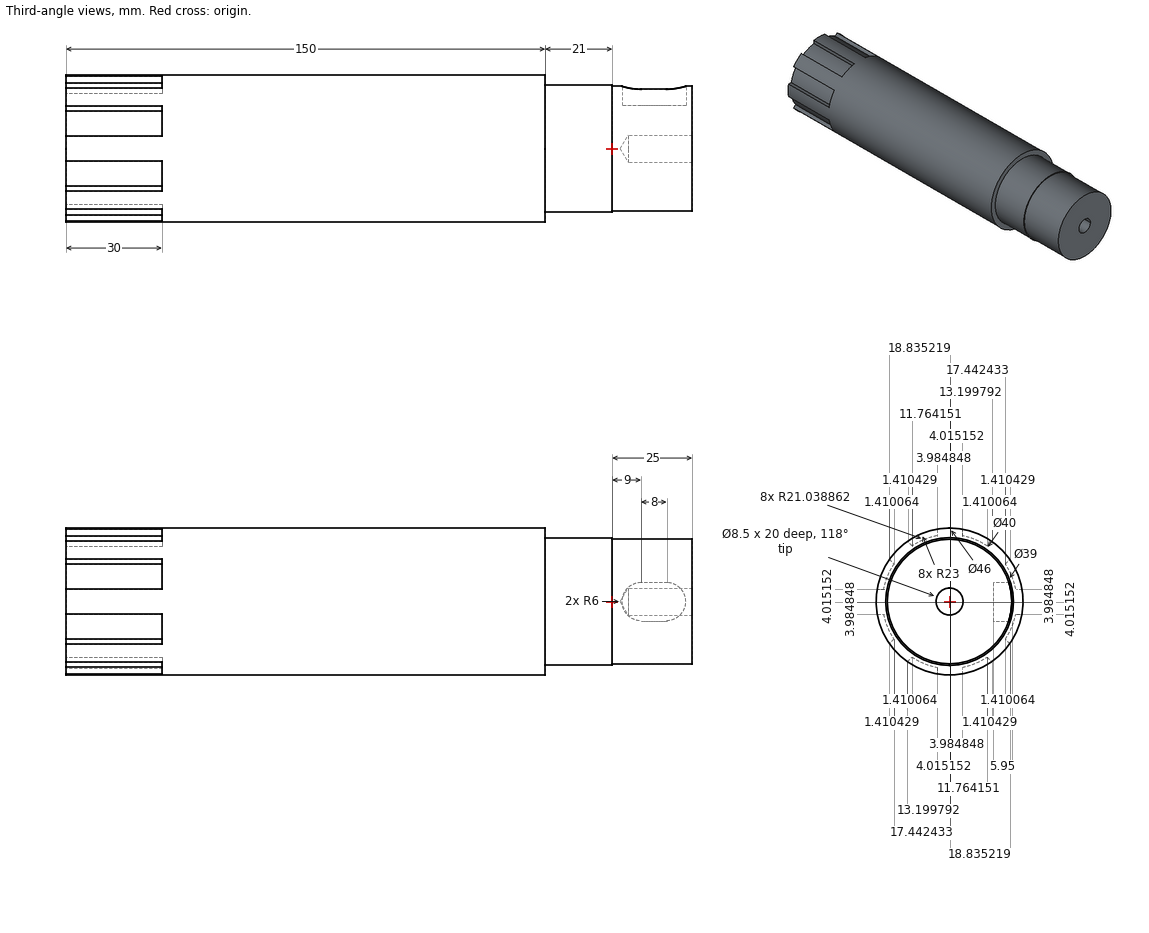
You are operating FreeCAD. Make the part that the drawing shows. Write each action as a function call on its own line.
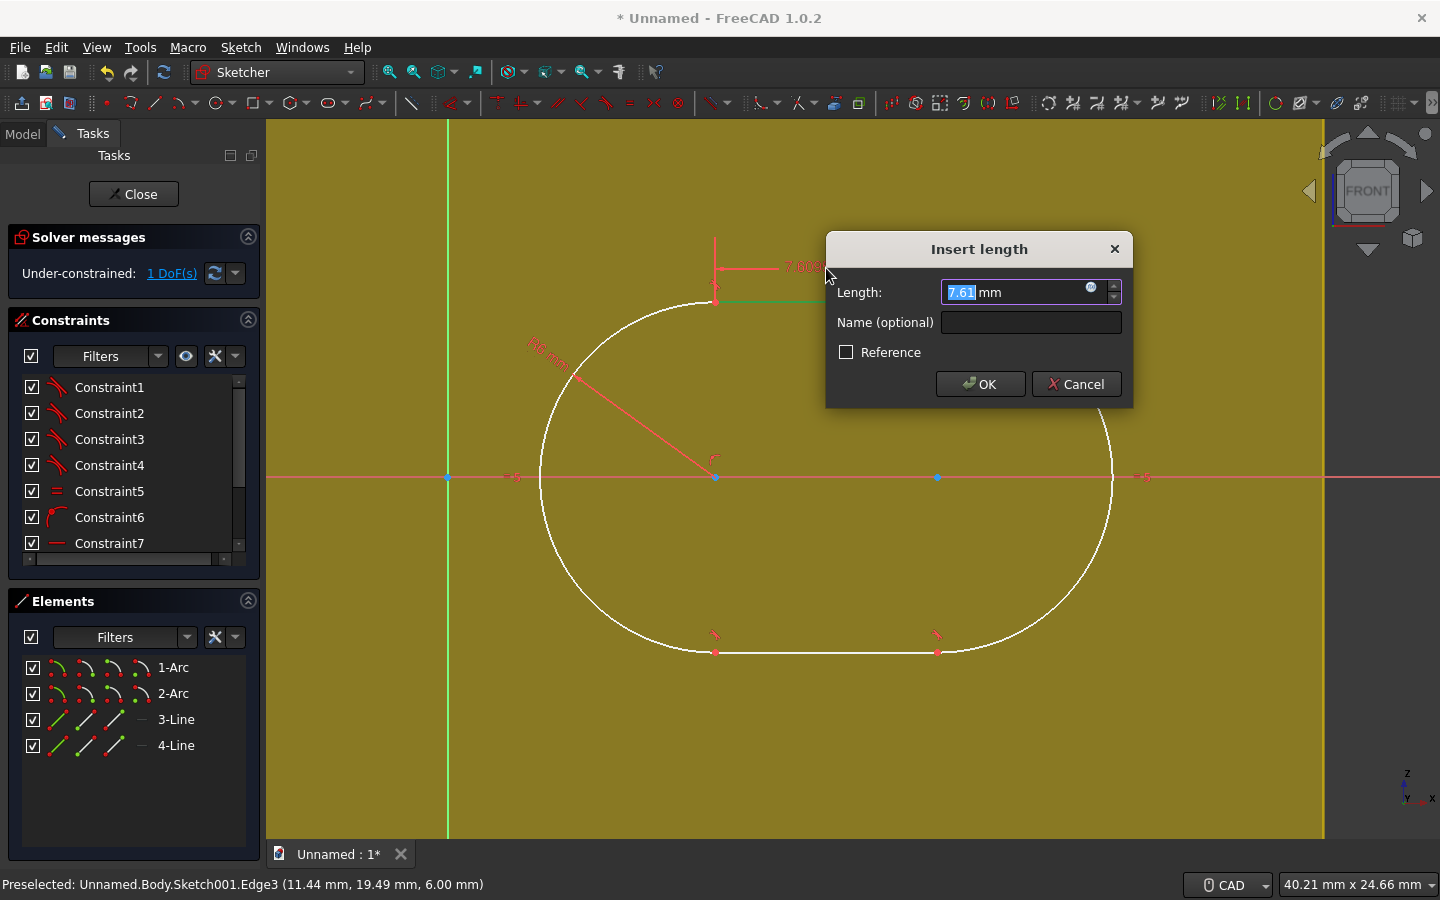
text(8)
key(Return)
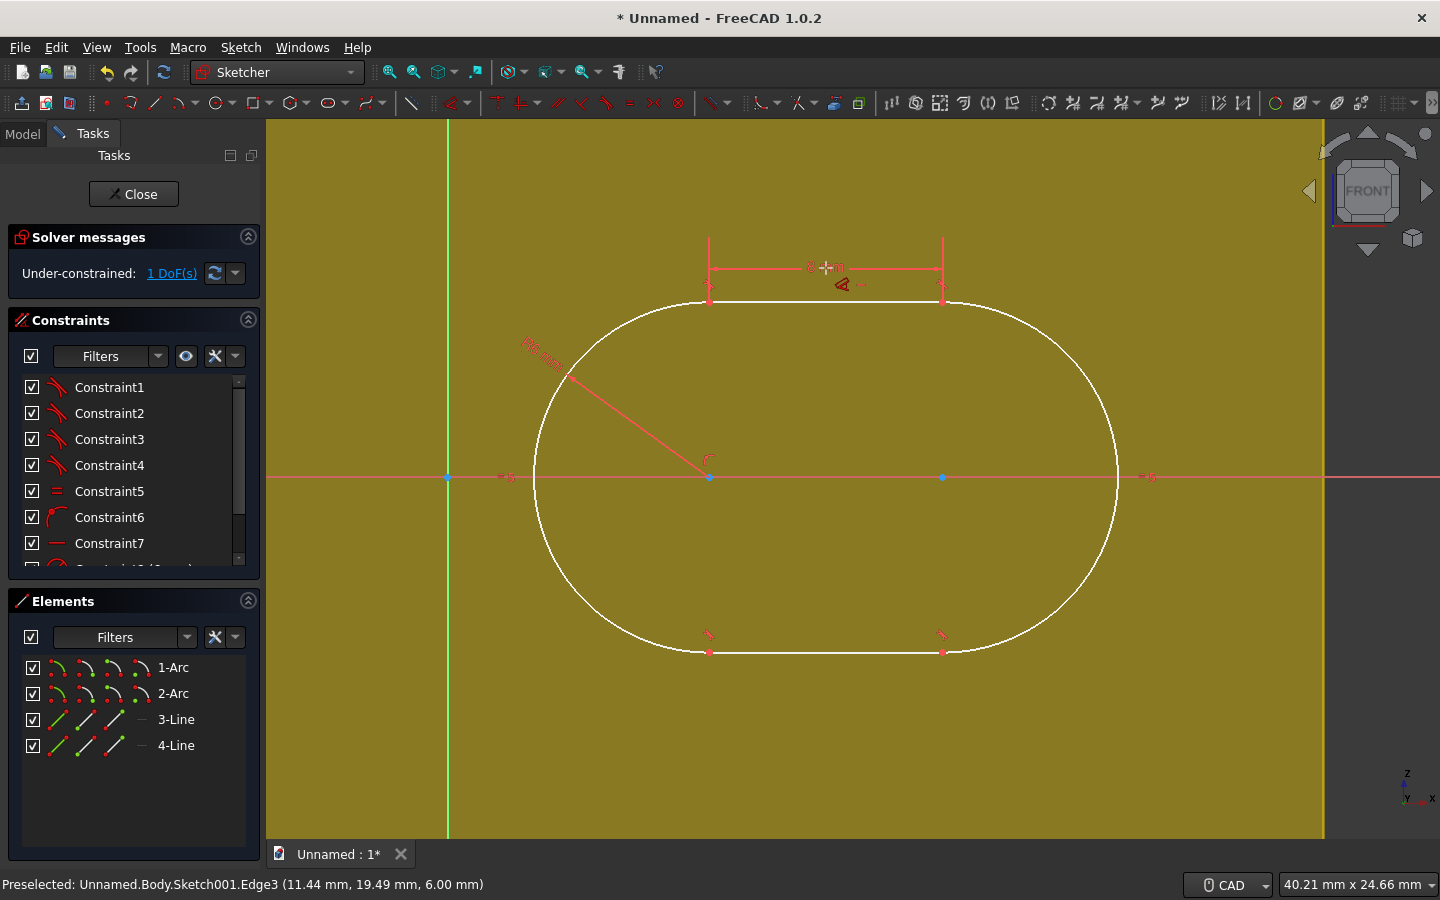
click(709, 302)
click(579, 268)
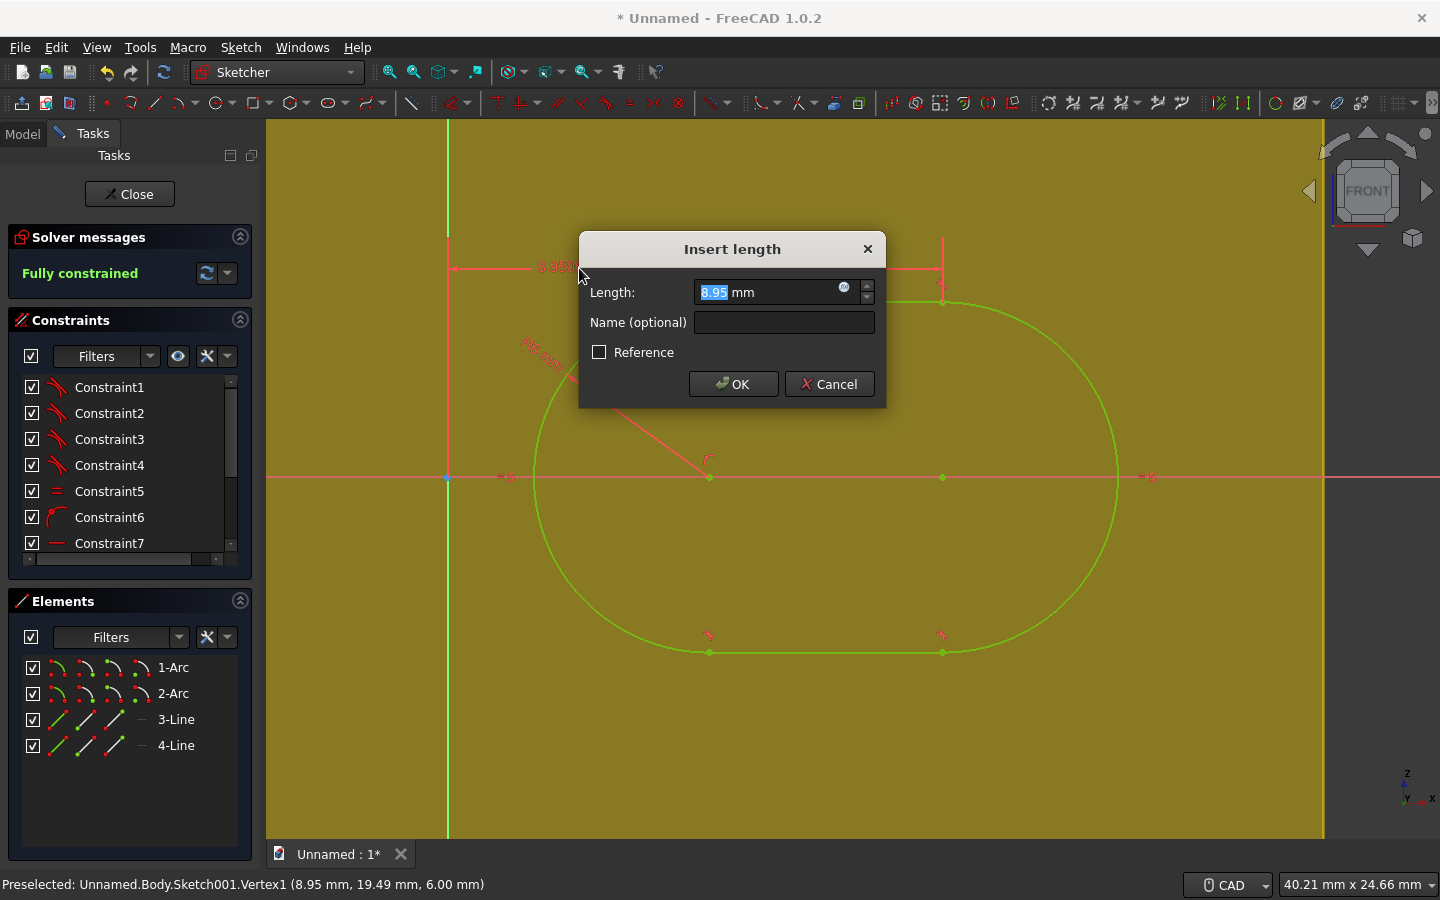
text(9)
key(Return)
key(Escape)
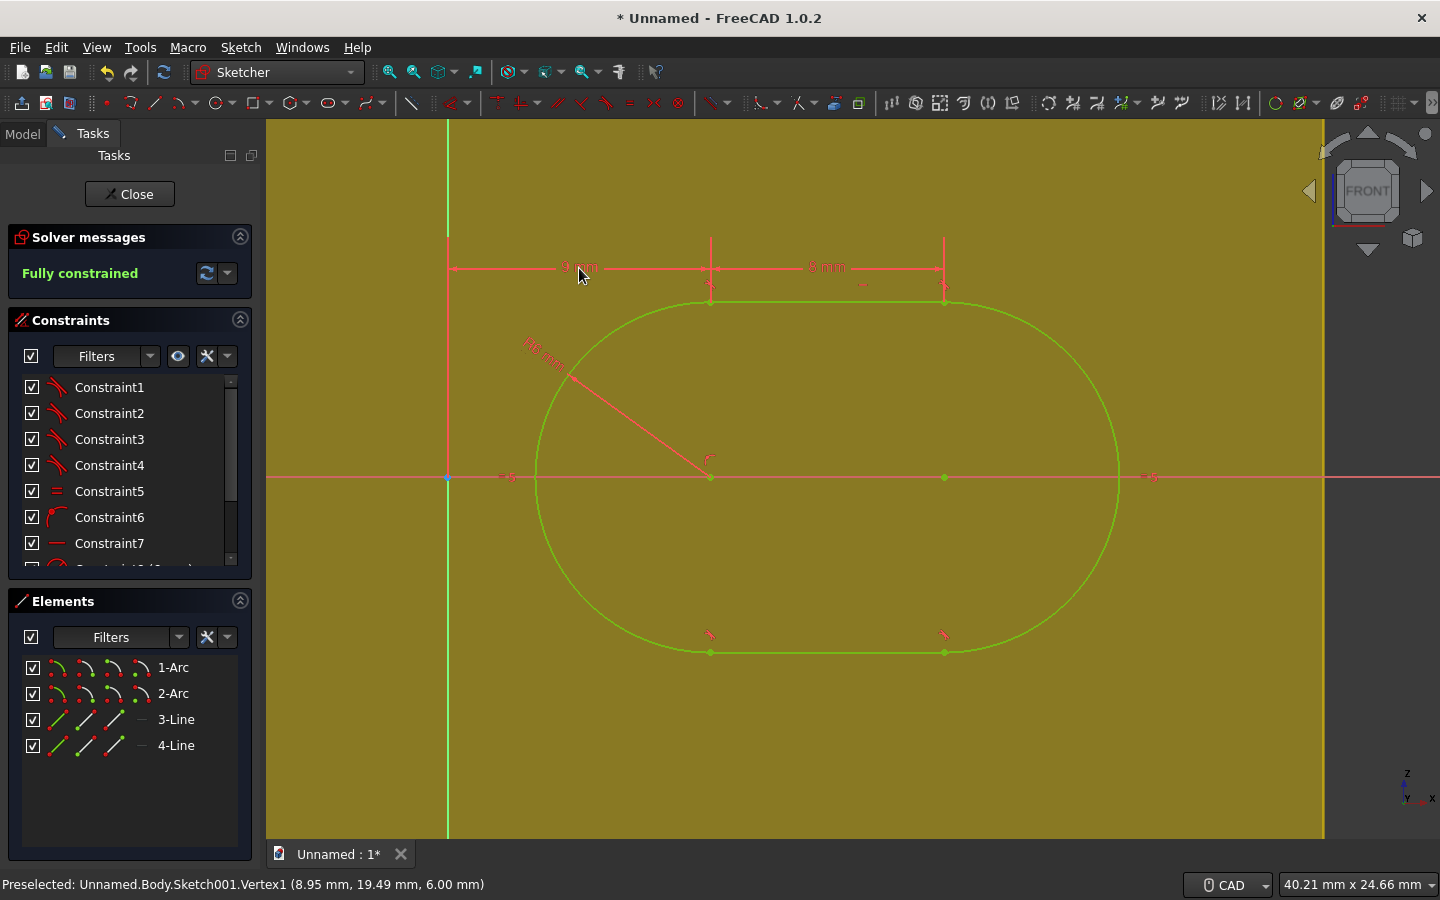
click(130, 194)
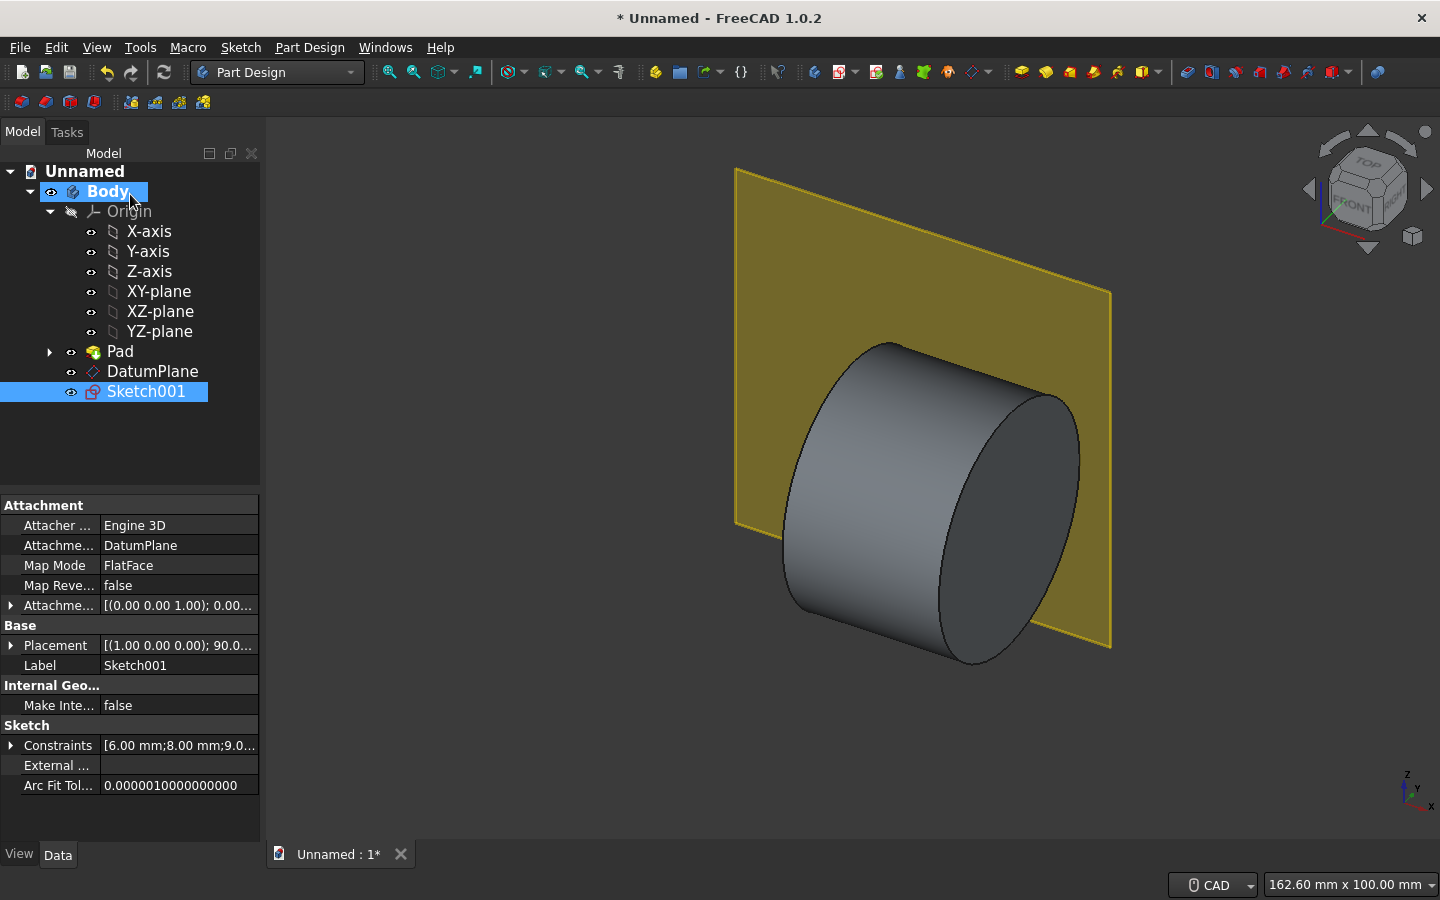
click(1188, 72)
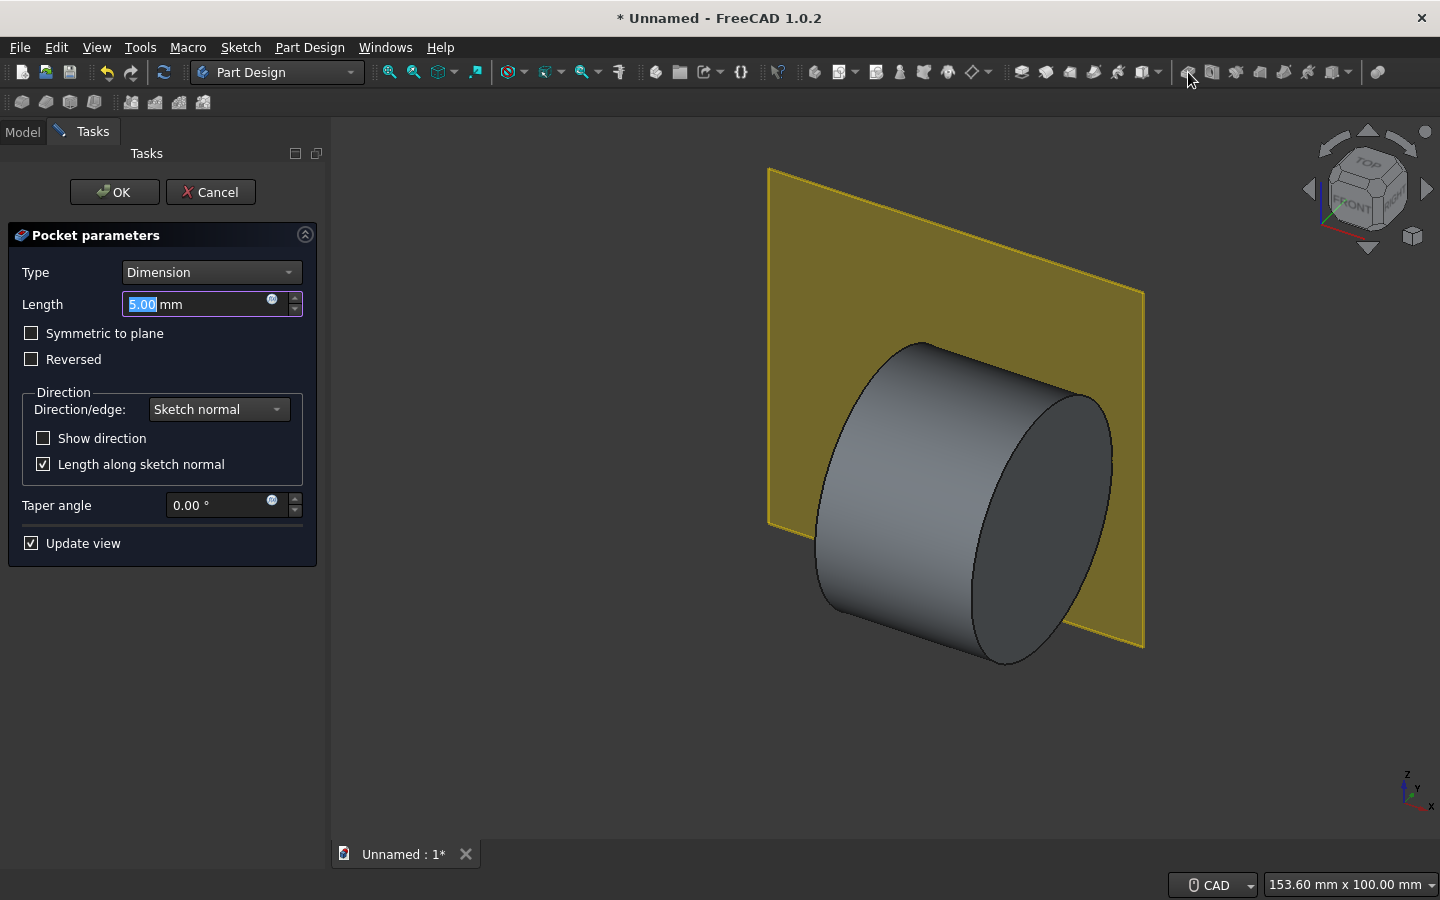
text(5.95)
key(Tab)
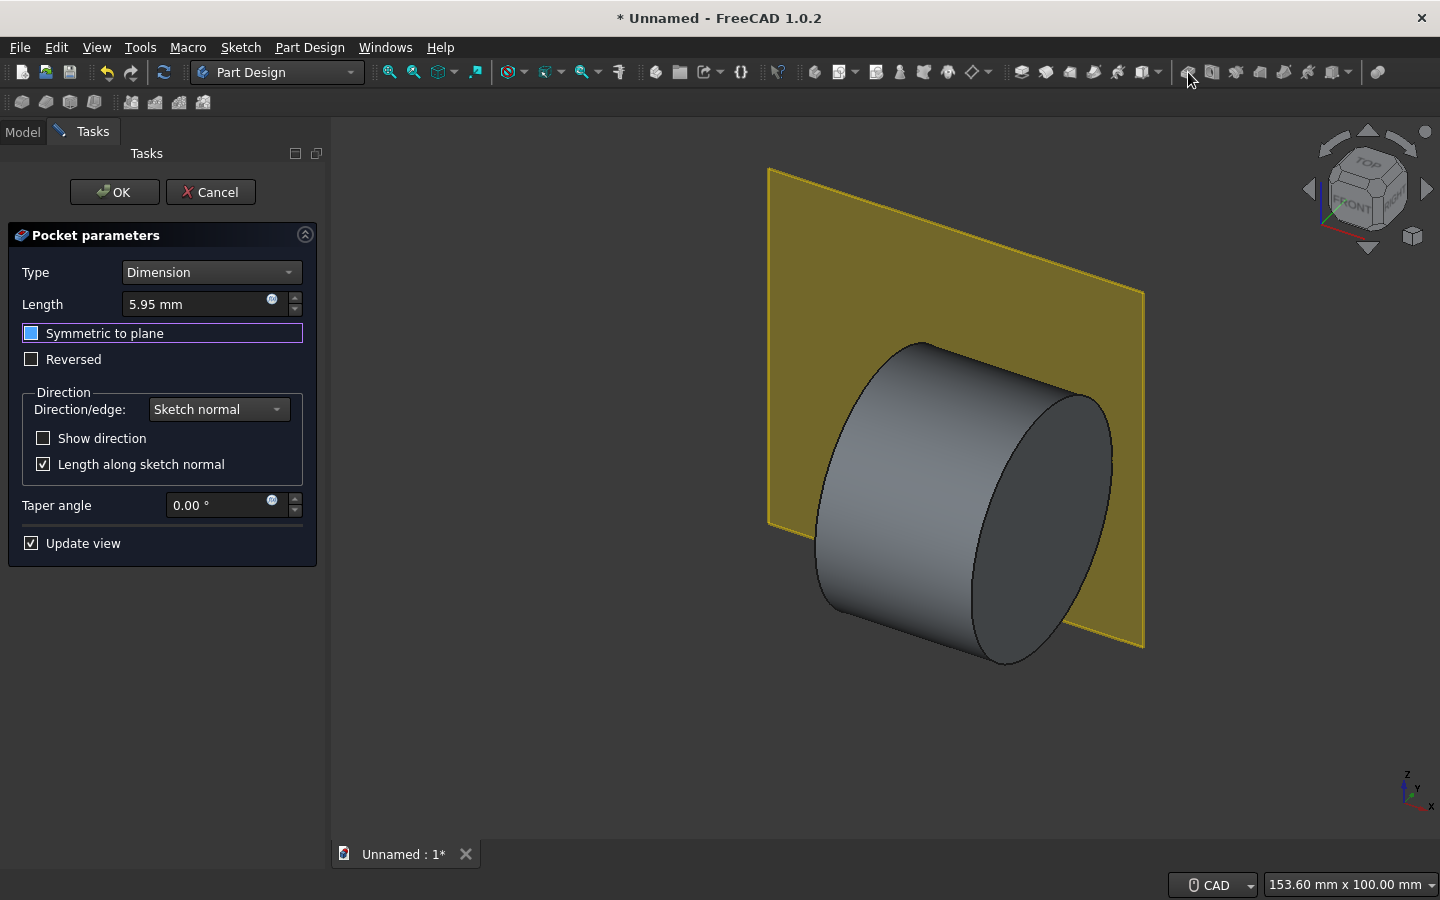
click(30, 359)